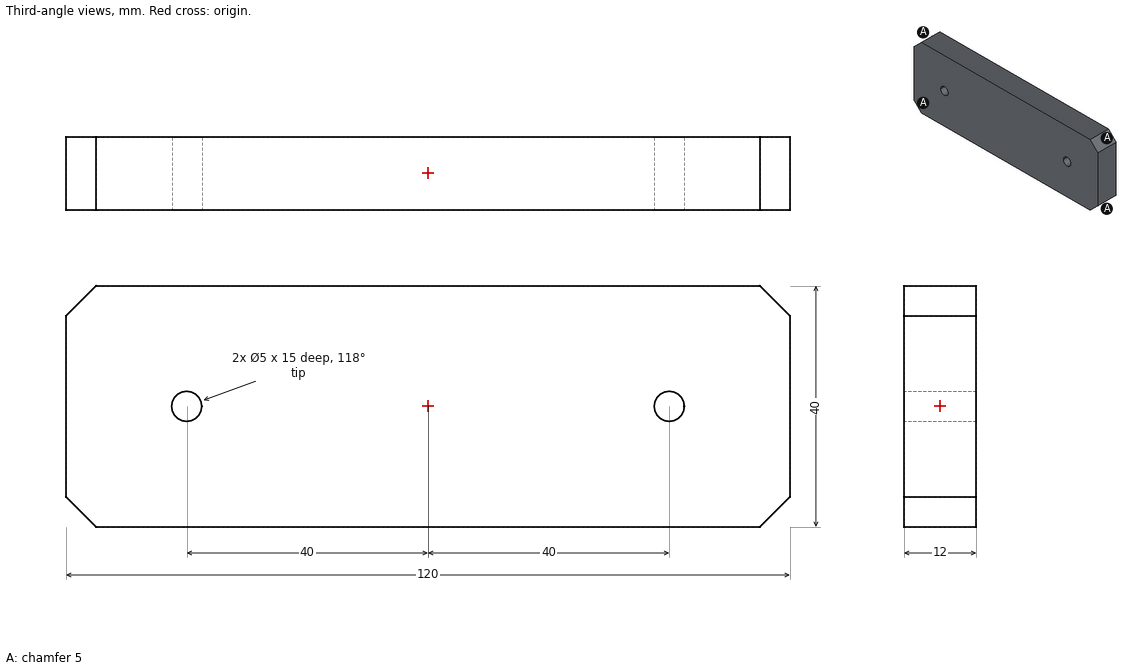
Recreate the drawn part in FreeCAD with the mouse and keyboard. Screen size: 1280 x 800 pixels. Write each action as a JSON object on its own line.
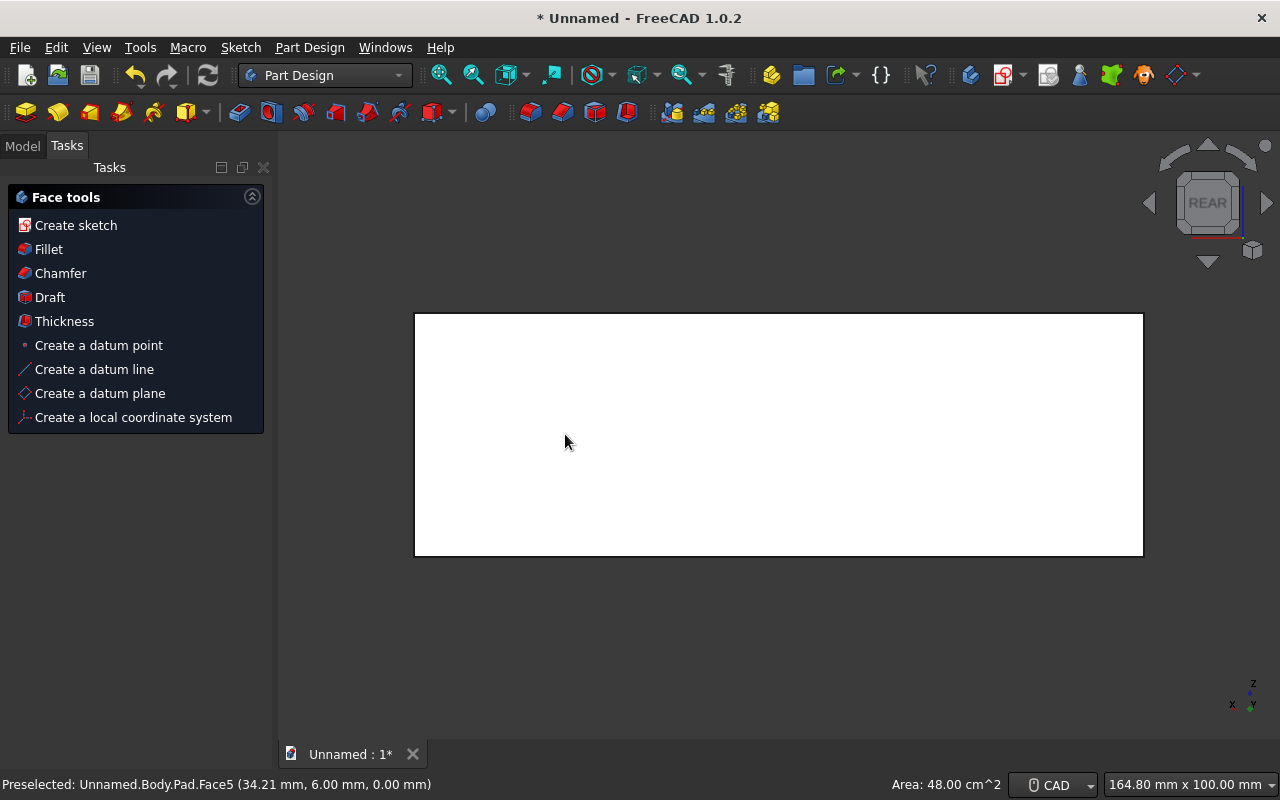
{"action": "left_click", "coordinate": [1004, 76]}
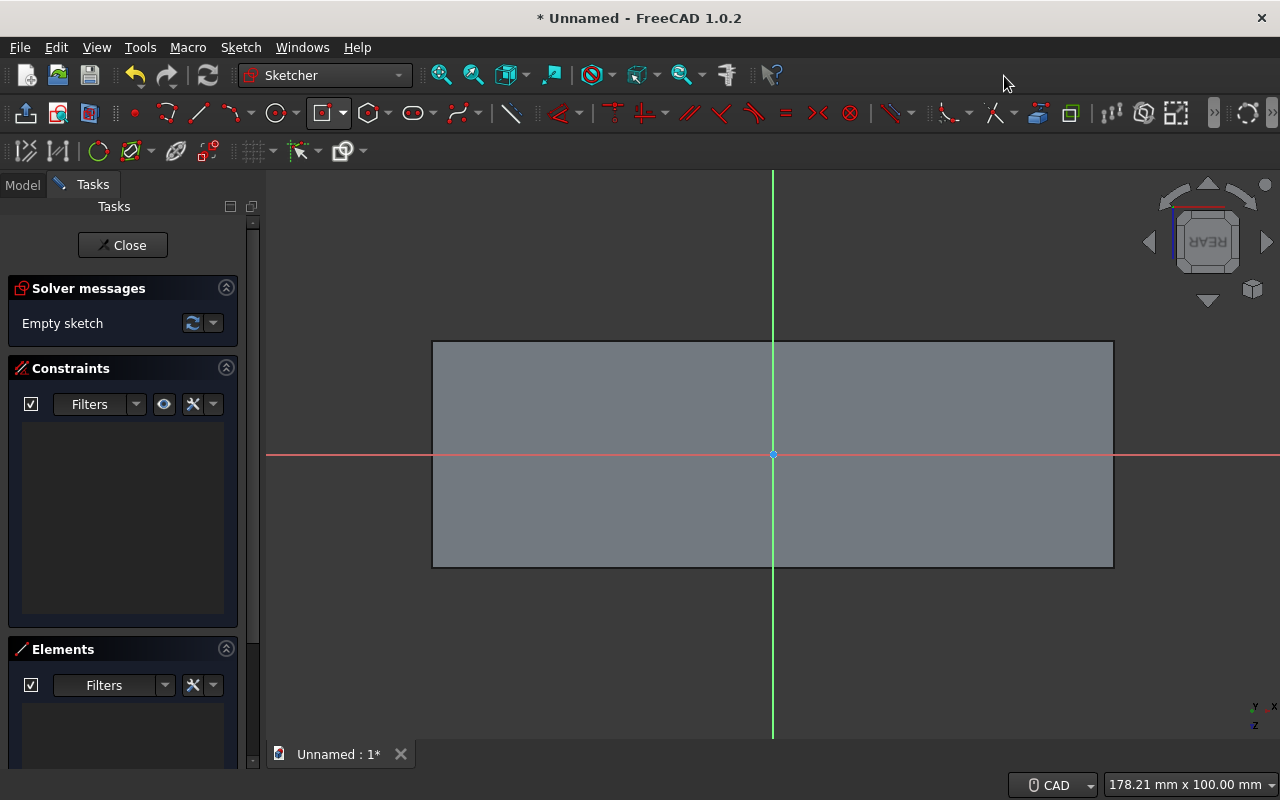
{"action": "left_click", "coordinate": [276, 114]}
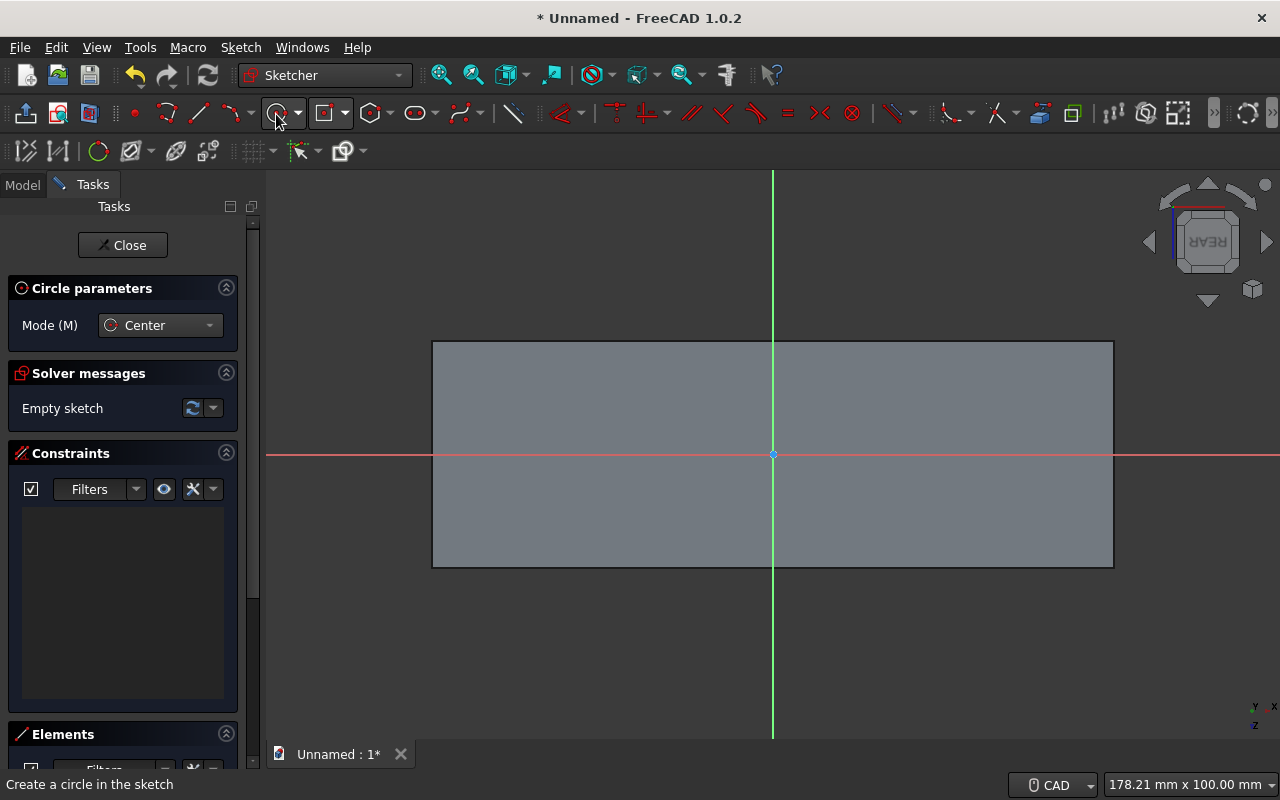
{"action": "scroll", "coordinate": [545, 455], "scroll_direction": "up", "scroll_amount": 3}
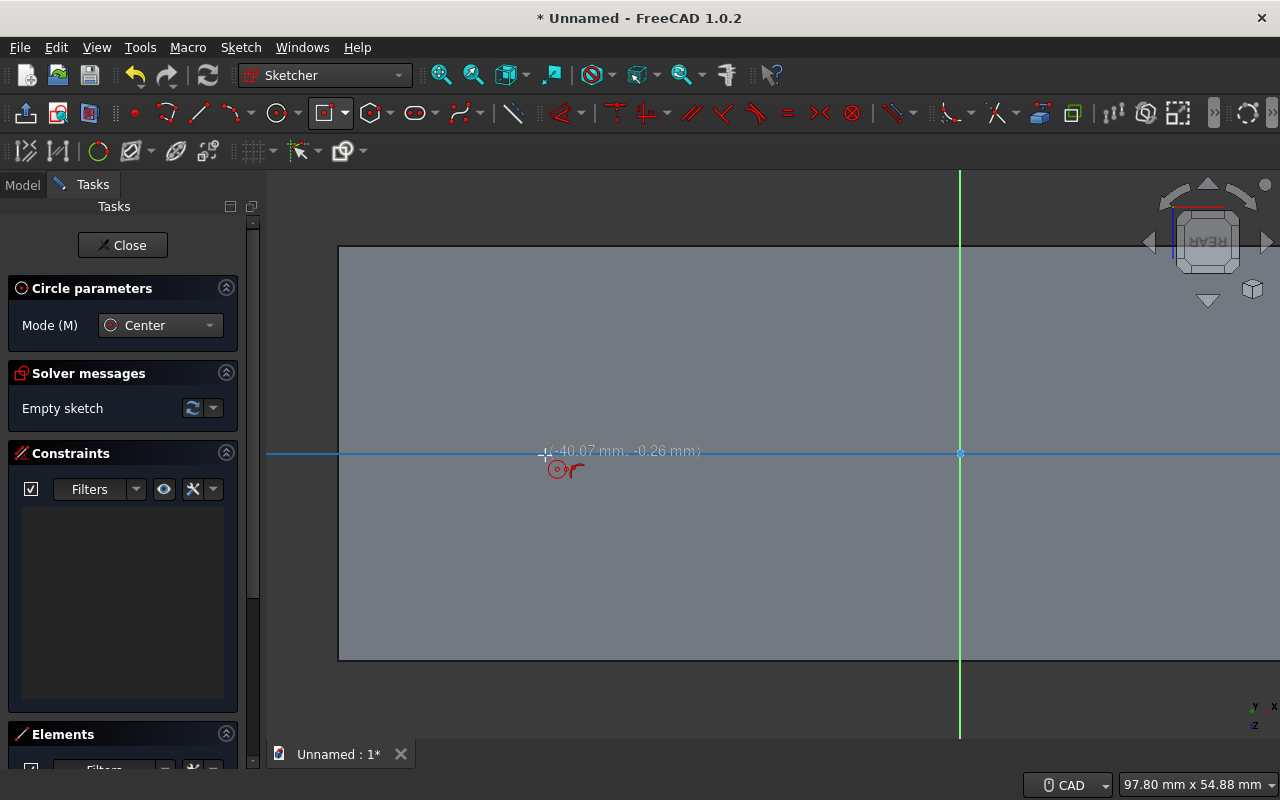
{"action": "left_click", "coordinate": [546, 454]}
{"action": "left_click", "coordinate": [564, 435]}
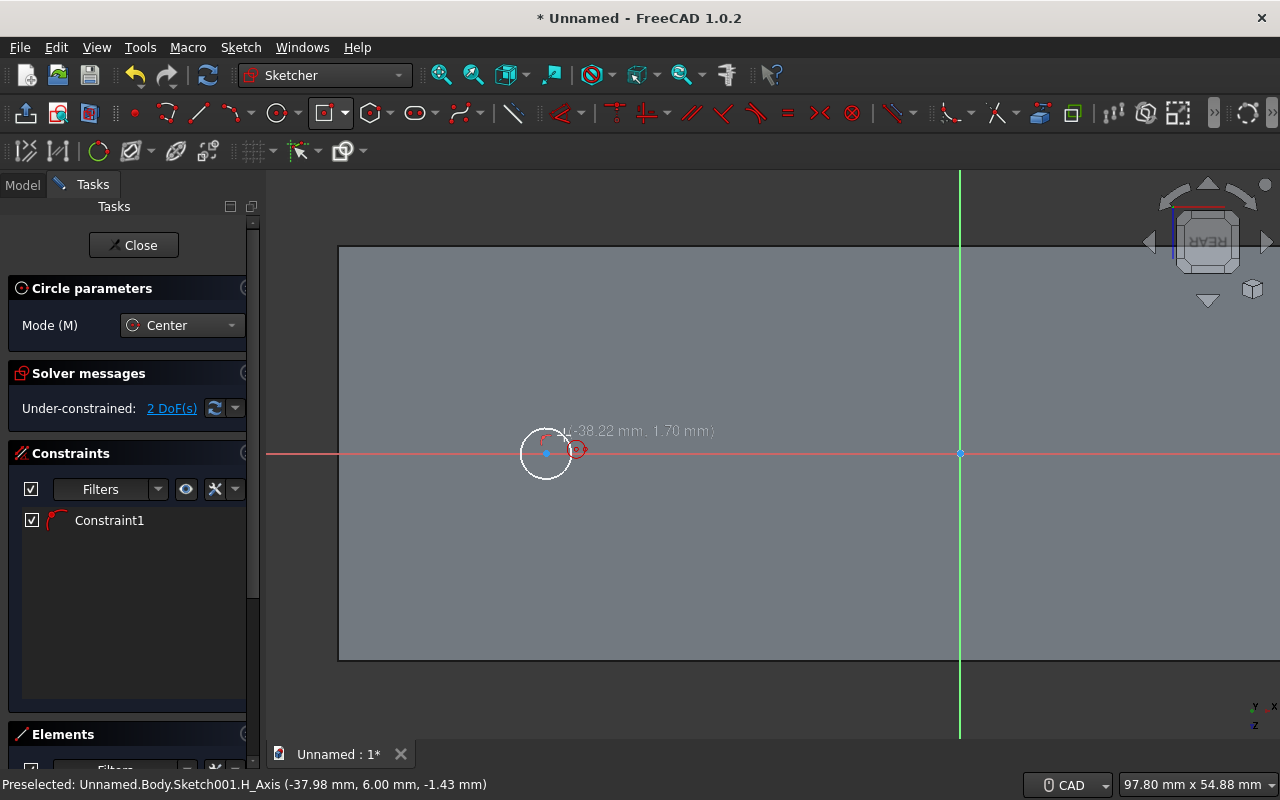
{"action": "scroll", "coordinate": [294, 456], "scroll_direction": "down", "scroll_amount": 2}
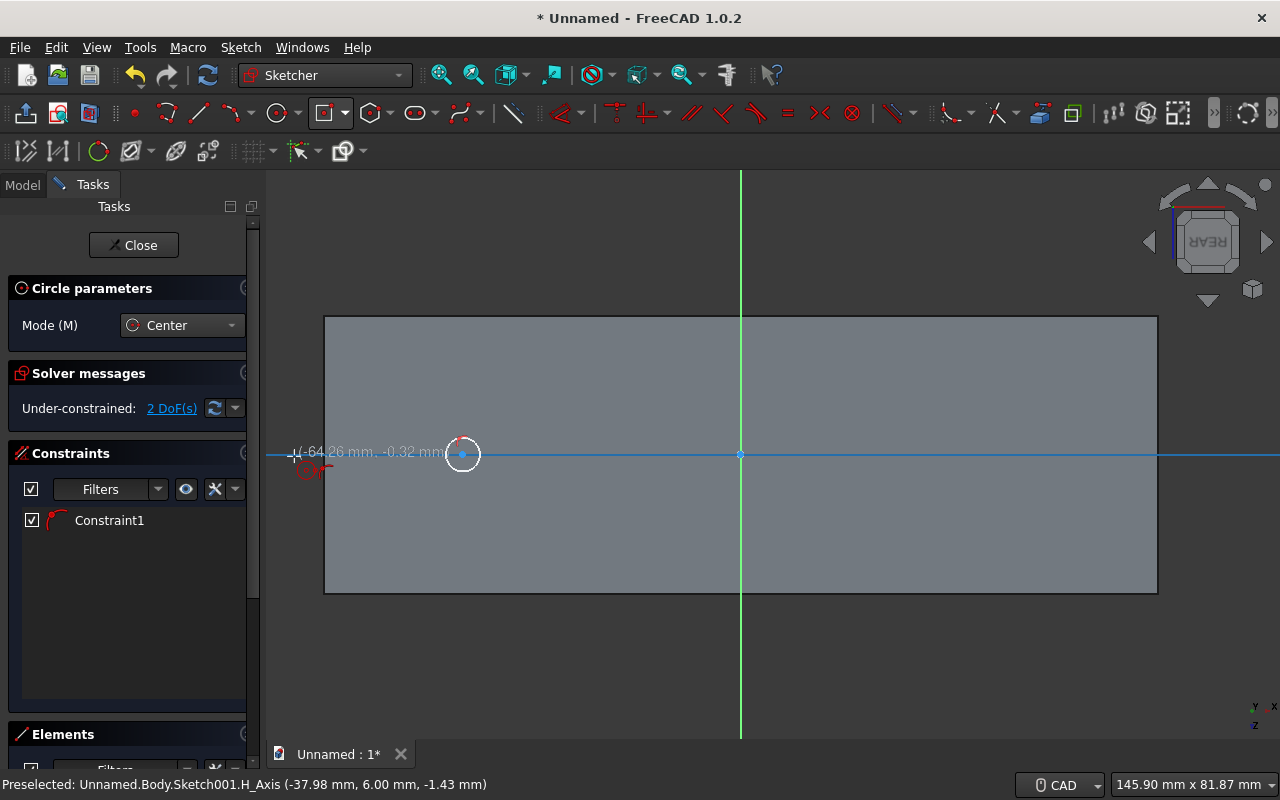
{"action": "scroll", "coordinate": [1019, 455], "scroll_direction": "up", "scroll_amount": 2}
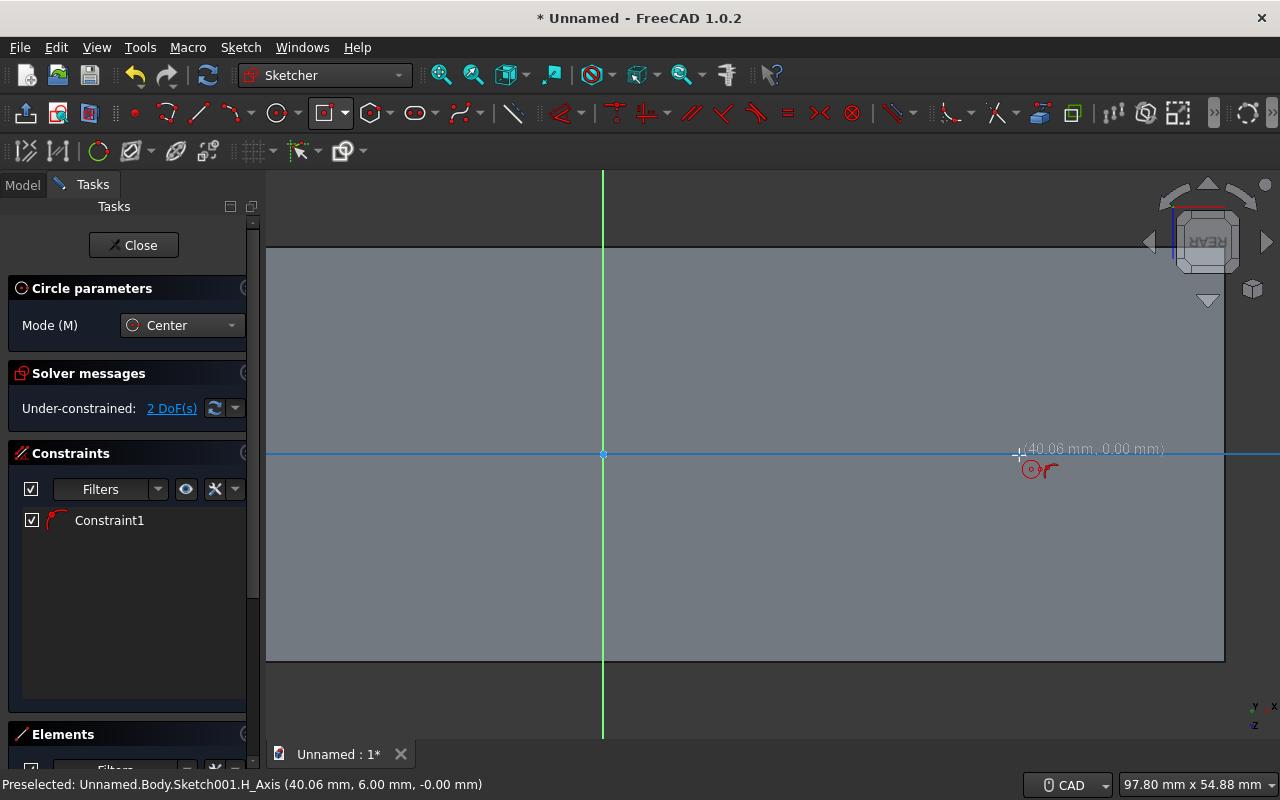
{"action": "left_click", "coordinate": [1018, 454]}
{"action": "left_click", "coordinate": [1036, 436]}
{"action": "key", "text": "Escape"}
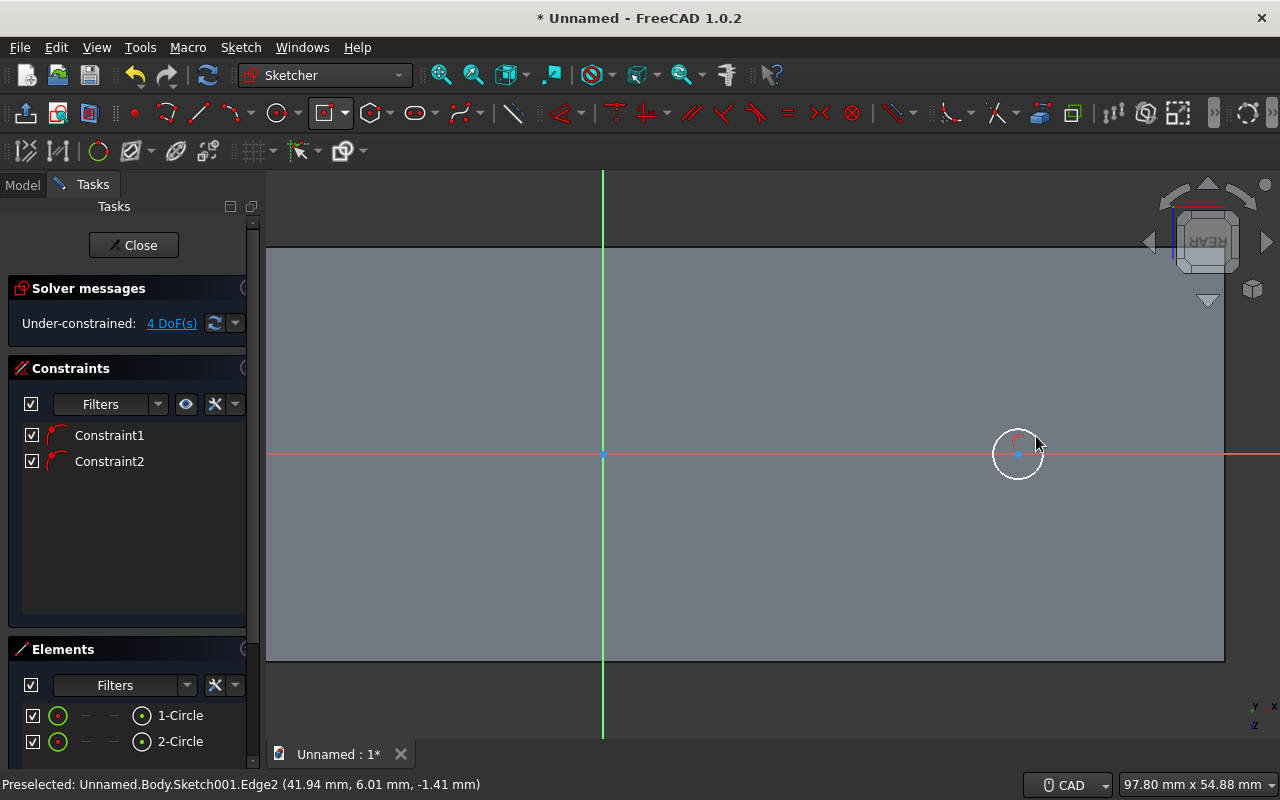
{"action": "scroll", "coordinate": [910, 455], "scroll_direction": "down", "scroll_amount": 2}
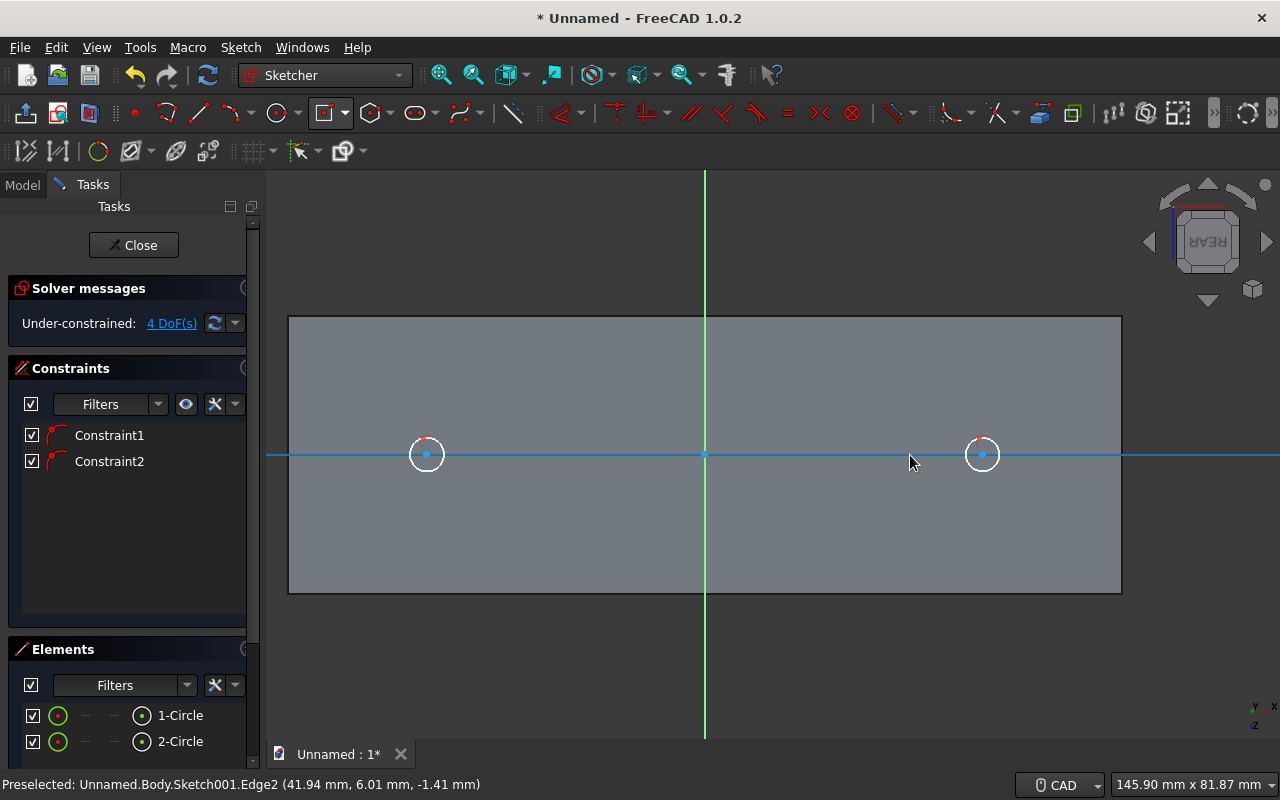
{"action": "left_click", "coordinate": [439, 443]}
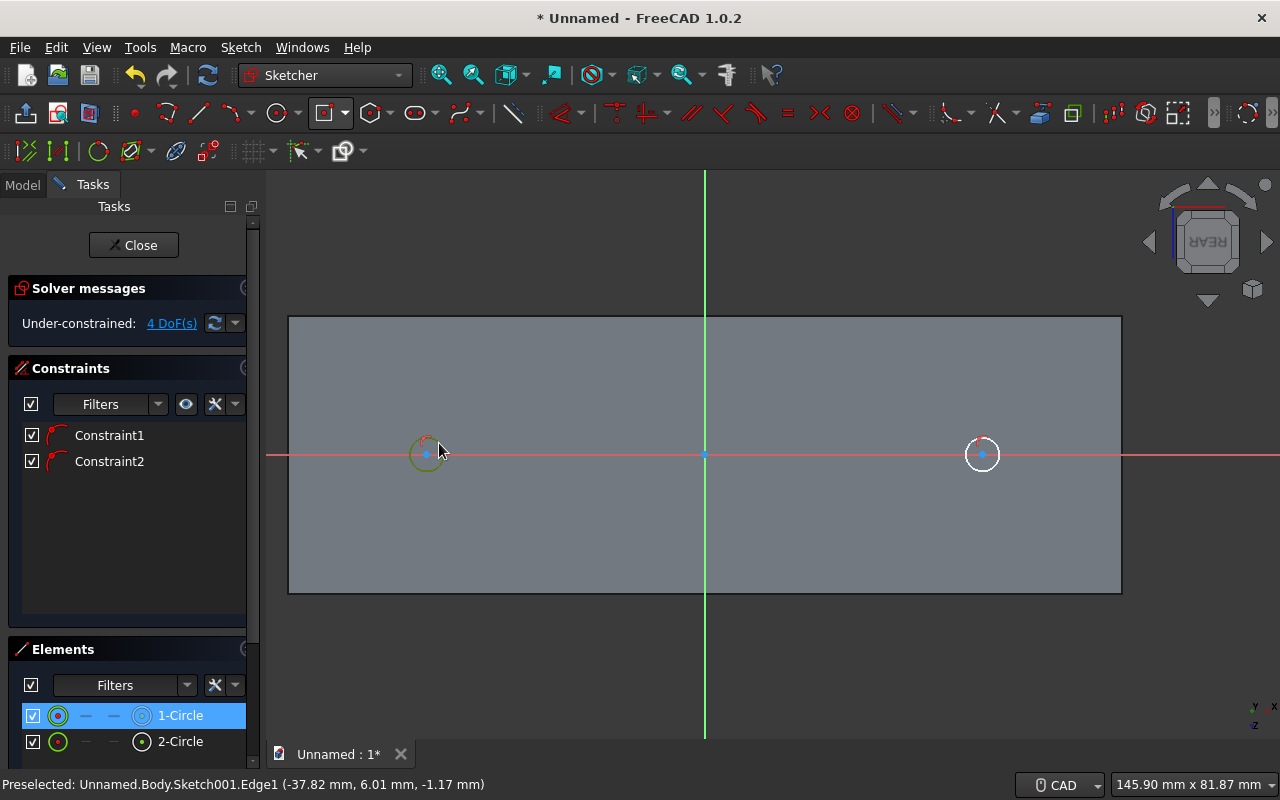
{"action": "left_click", "coordinate": [994, 443]}